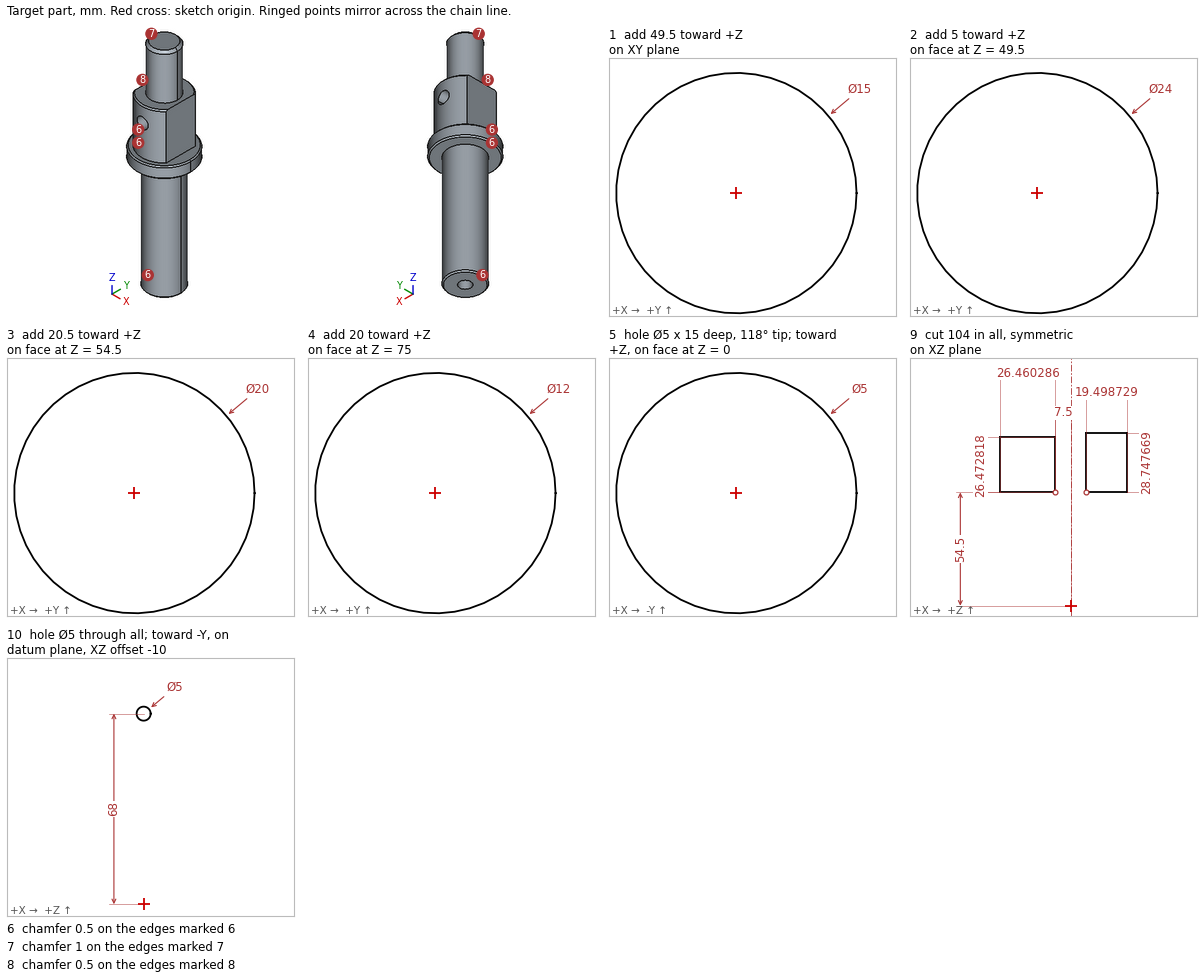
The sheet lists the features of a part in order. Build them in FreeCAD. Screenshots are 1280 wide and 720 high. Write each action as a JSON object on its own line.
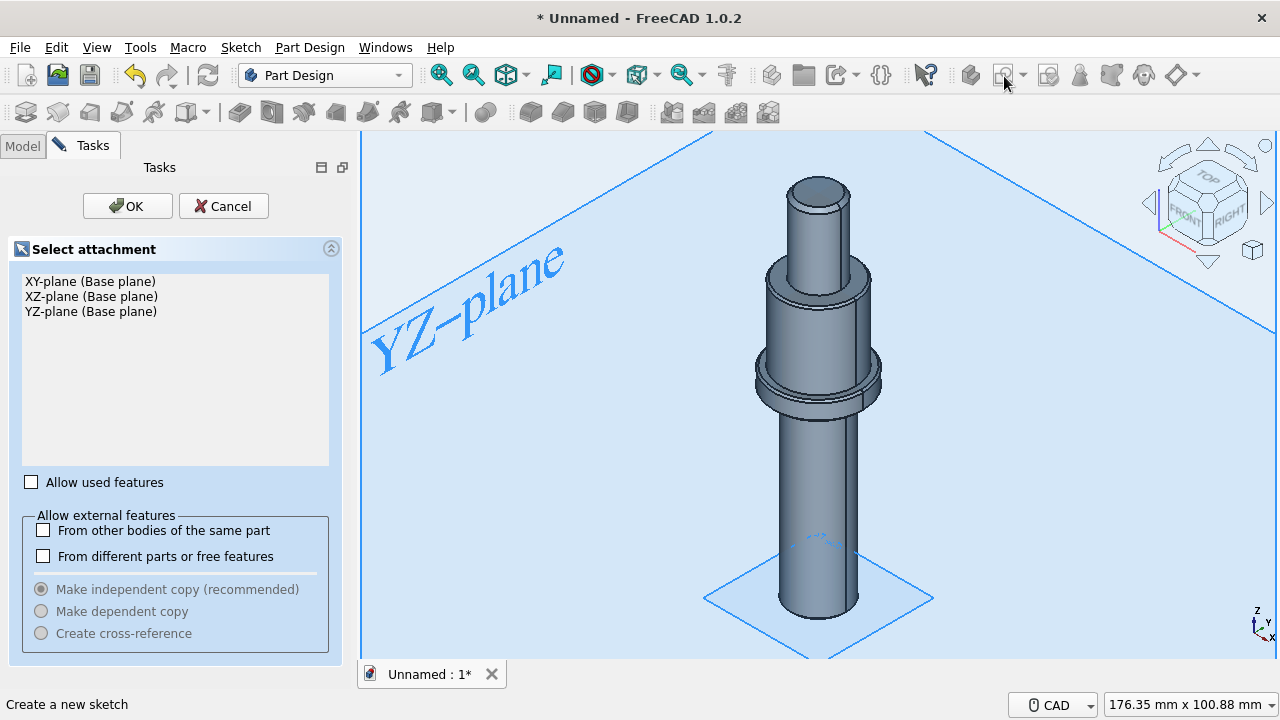
{"action": "left_click", "coordinate": [82, 296]}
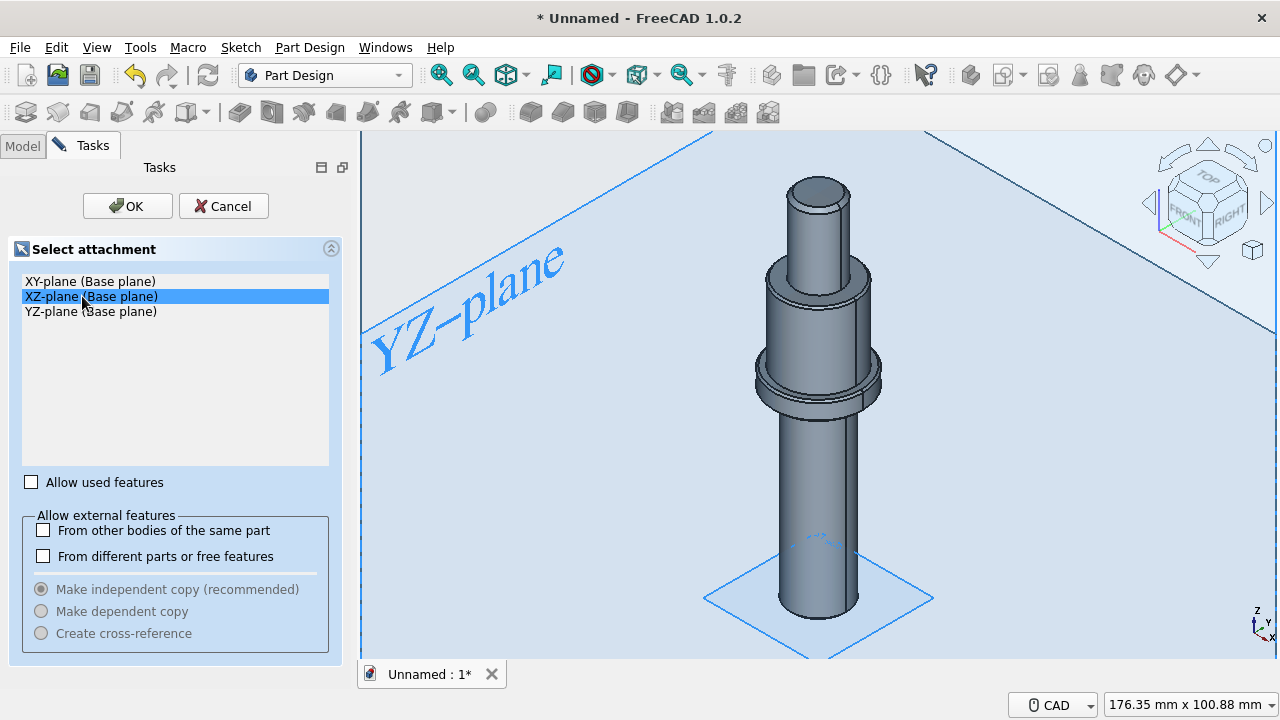
{"action": "left_click", "coordinate": [128, 206]}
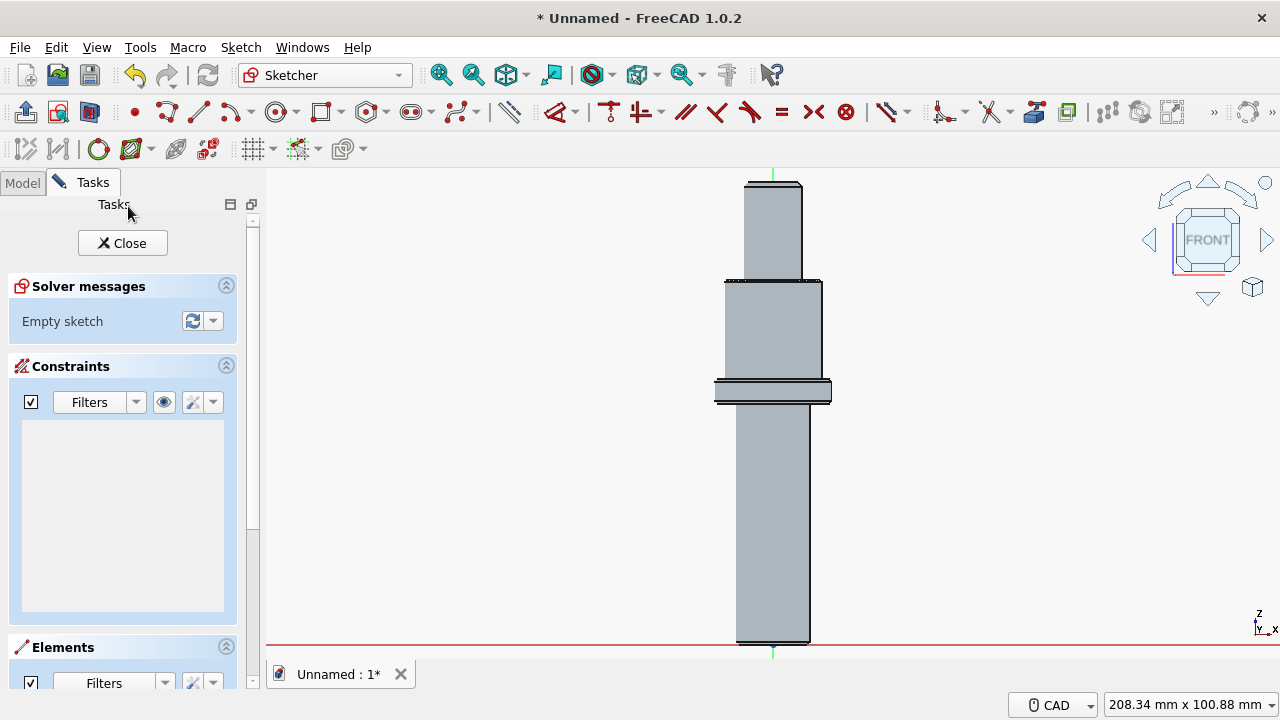
{"action": "key", "text": "q s"}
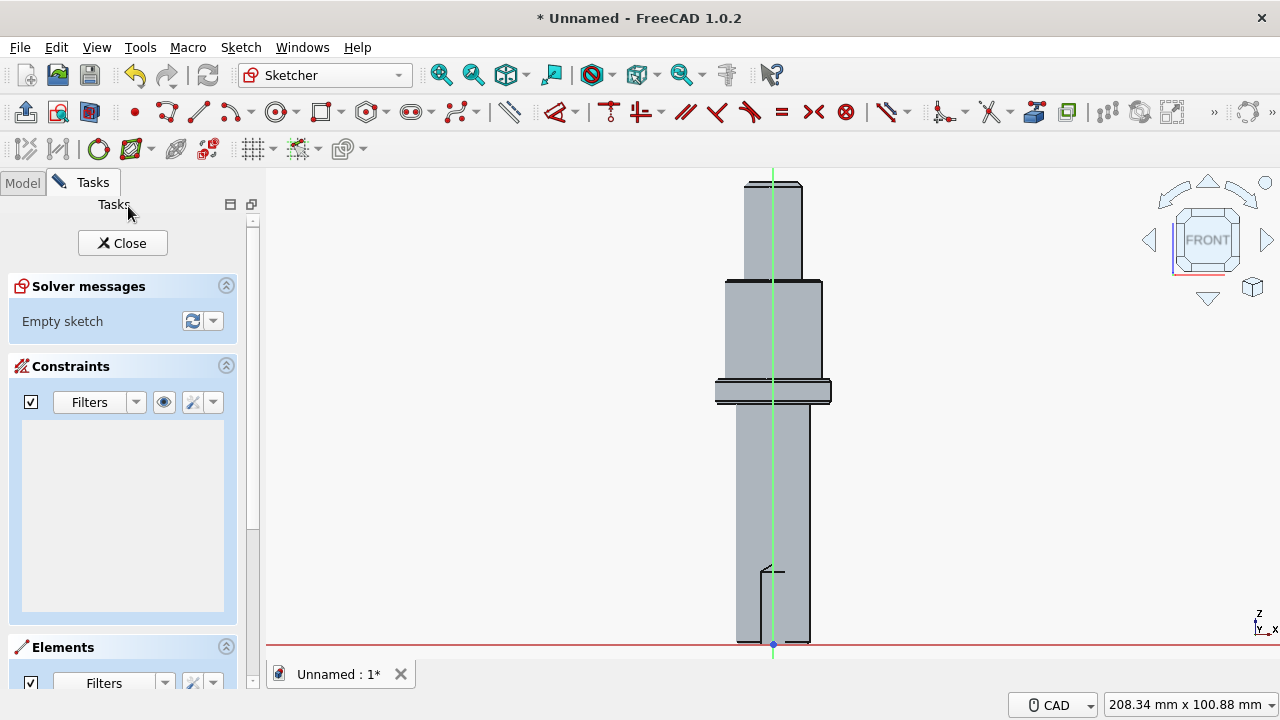
{"action": "scroll", "coordinate": [472, 284], "scroll_direction": "down", "scroll_amount": 1}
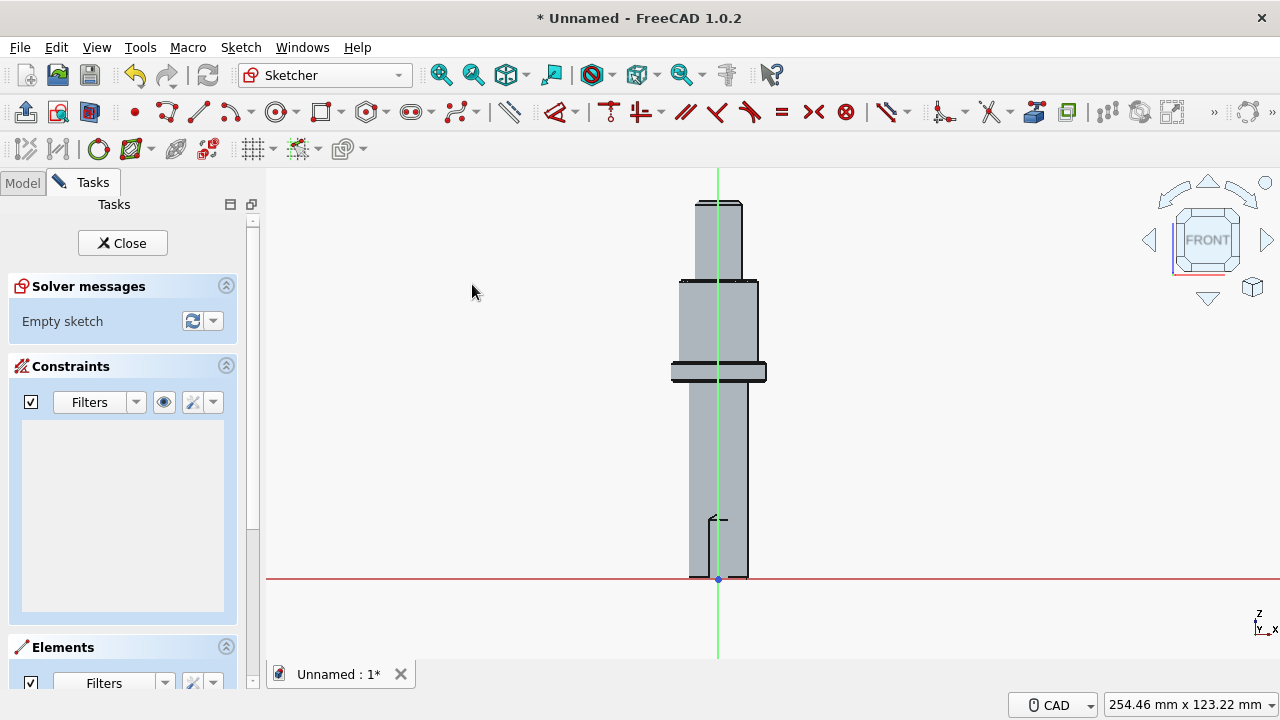
{"action": "key", "text": "g r"}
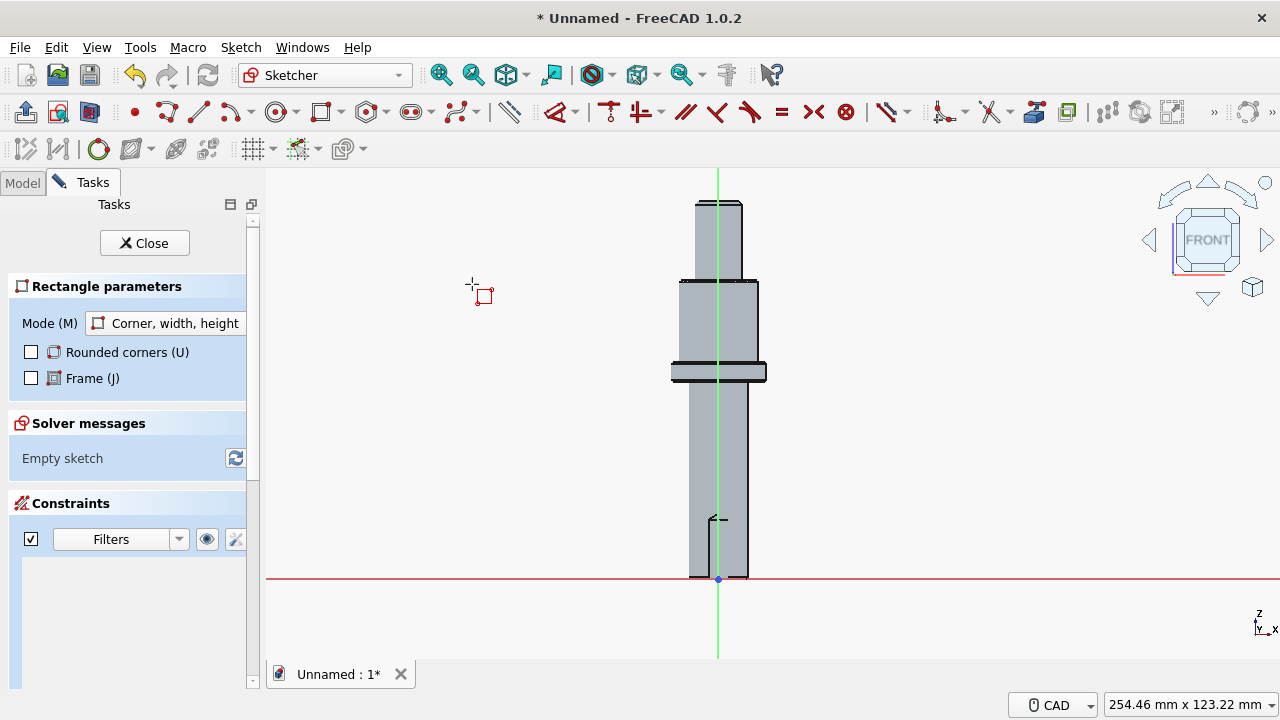
{"action": "left_click", "coordinate": [583, 257]}
{"action": "mouse_move", "coordinate": [689, 362]}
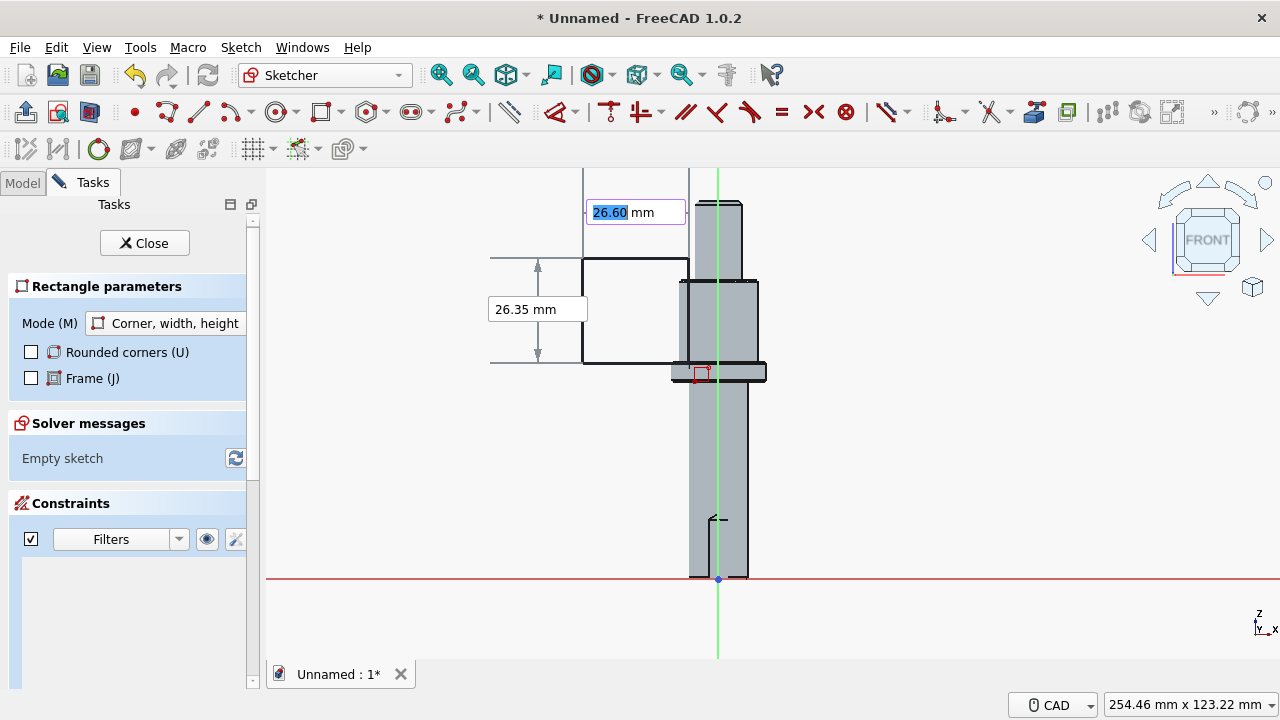
{"action": "type", "text": "26.460286"}
{"action": "key", "text": "Tab"}
{"action": "type", "text": "26.472818"}
{"action": "key", "text": "Return"}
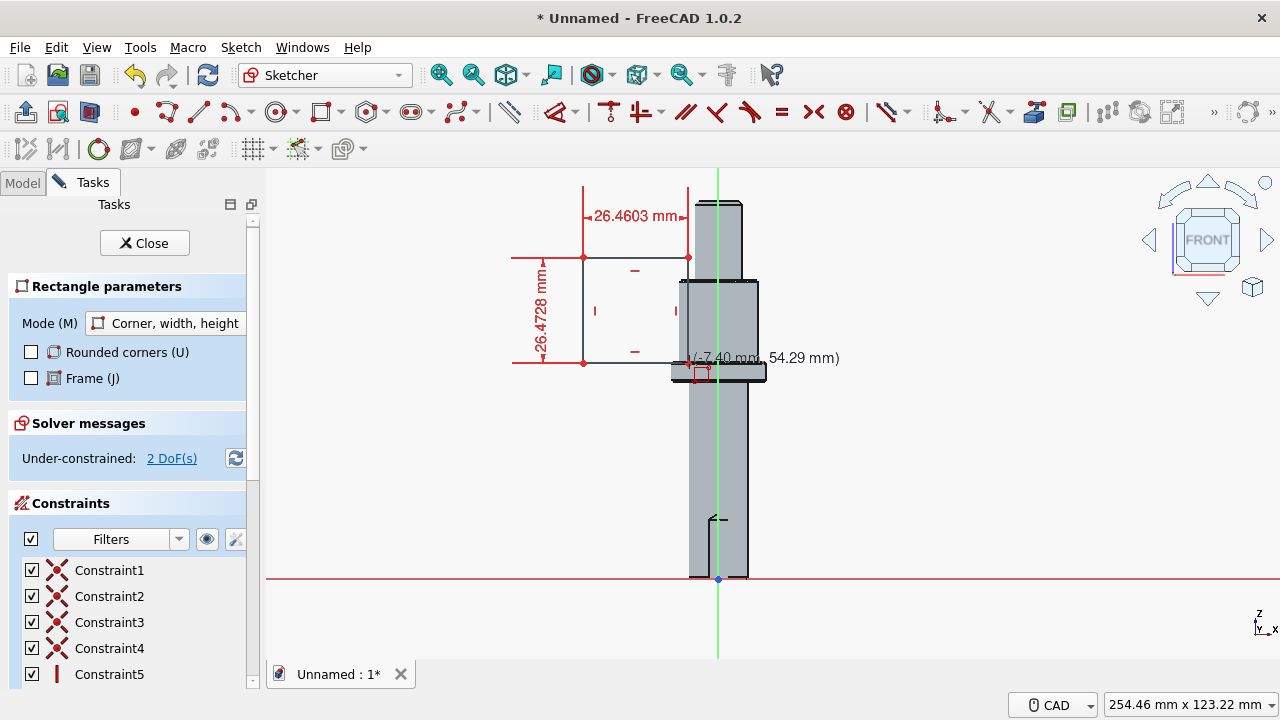
{"action": "left_click", "coordinate": [748, 248]}
{"action": "mouse_move", "coordinate": [826, 362]}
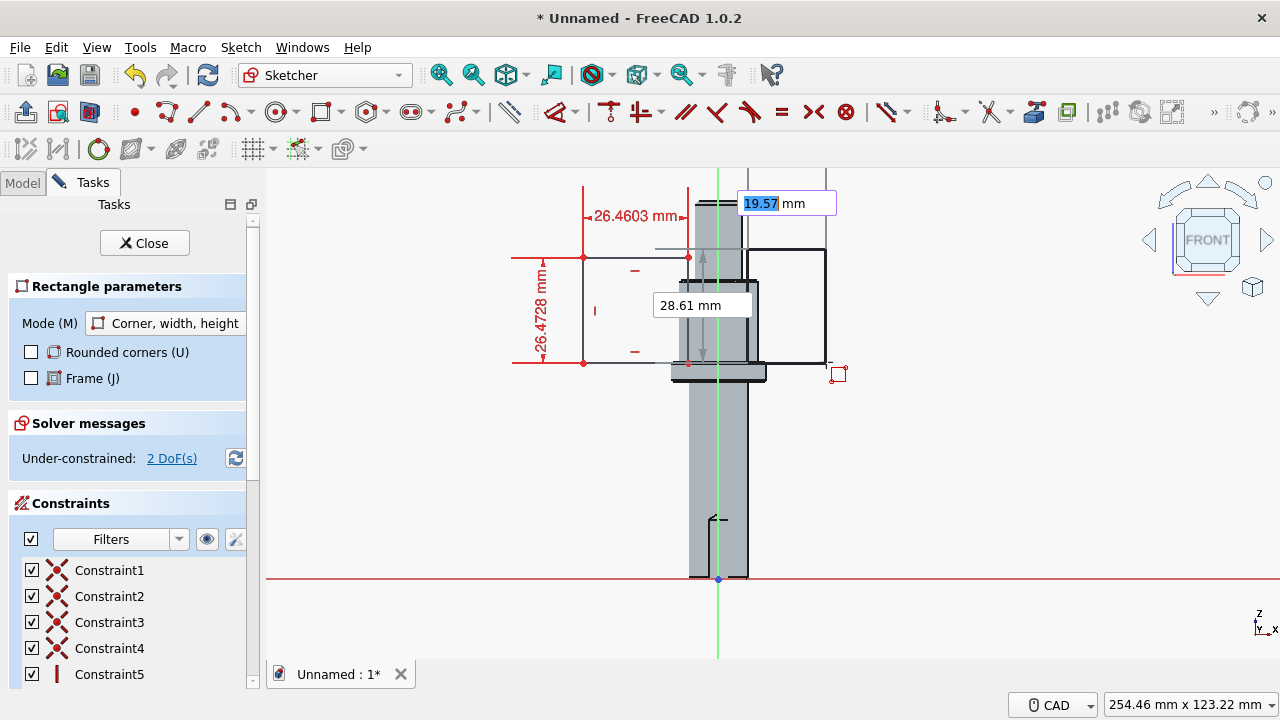
{"action": "type", "text": "19.498729"}
{"action": "key", "text": "Tab"}
{"action": "type", "text": "28.747669"}
{"action": "key", "text": "Return"}
{"action": "key", "text": "Escape"}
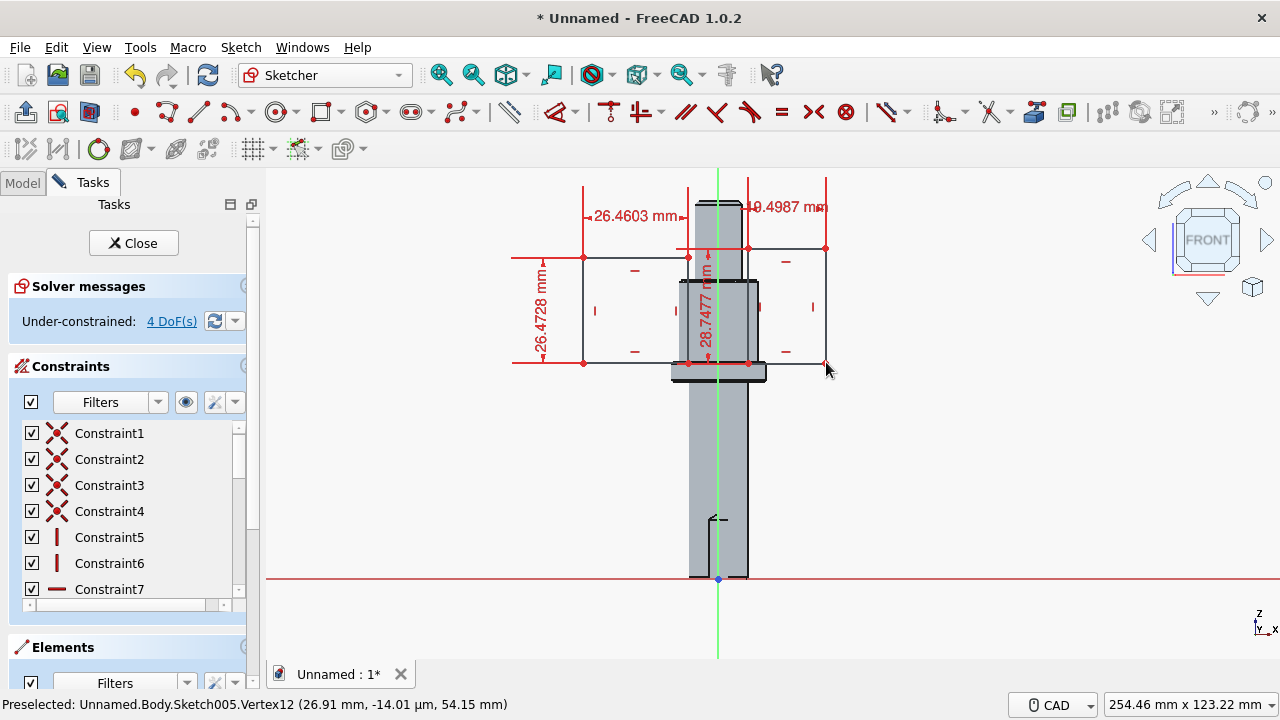
{"action": "left_click", "coordinate": [688, 363]}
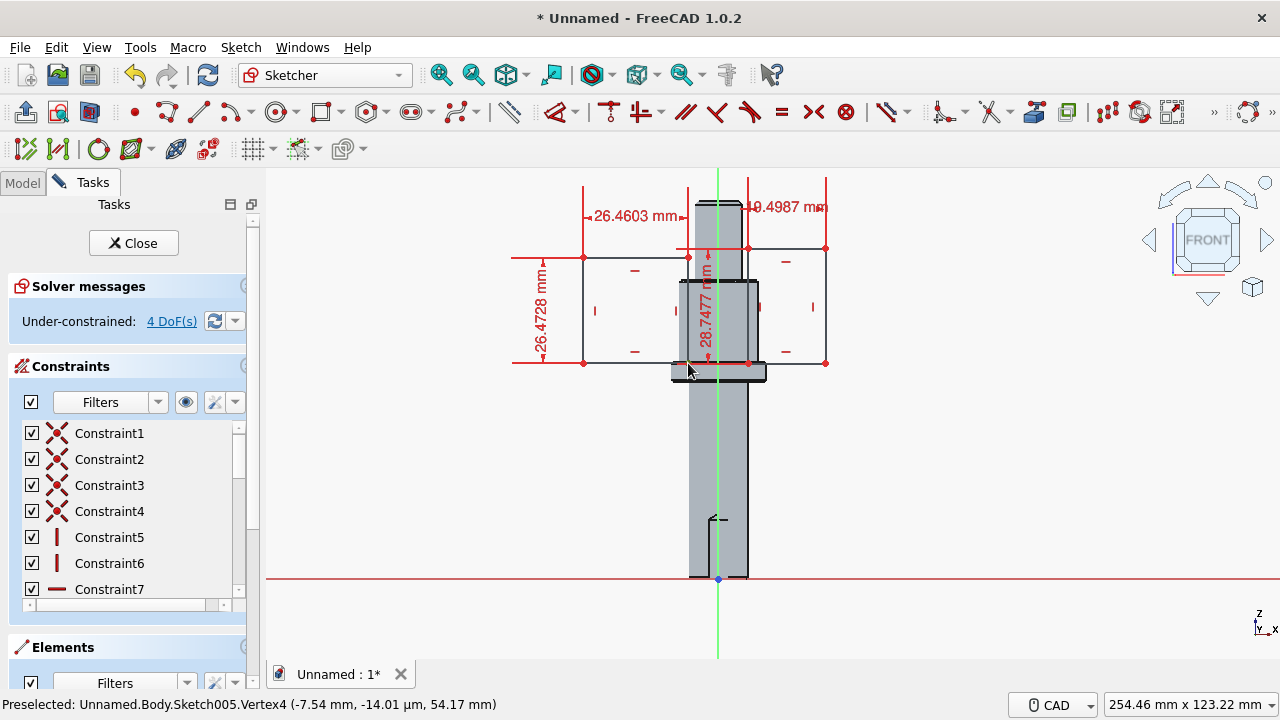
{"action": "left_click", "coordinate": [748, 364]}